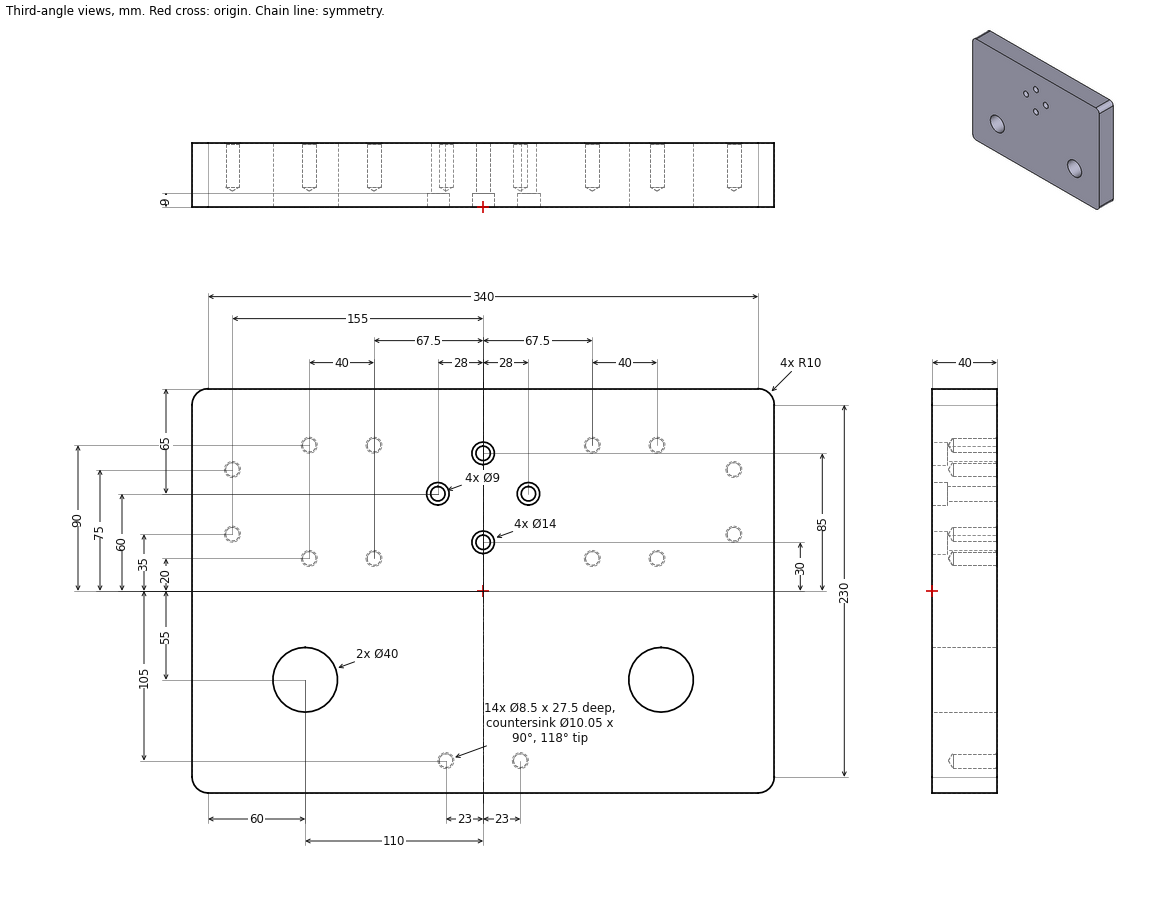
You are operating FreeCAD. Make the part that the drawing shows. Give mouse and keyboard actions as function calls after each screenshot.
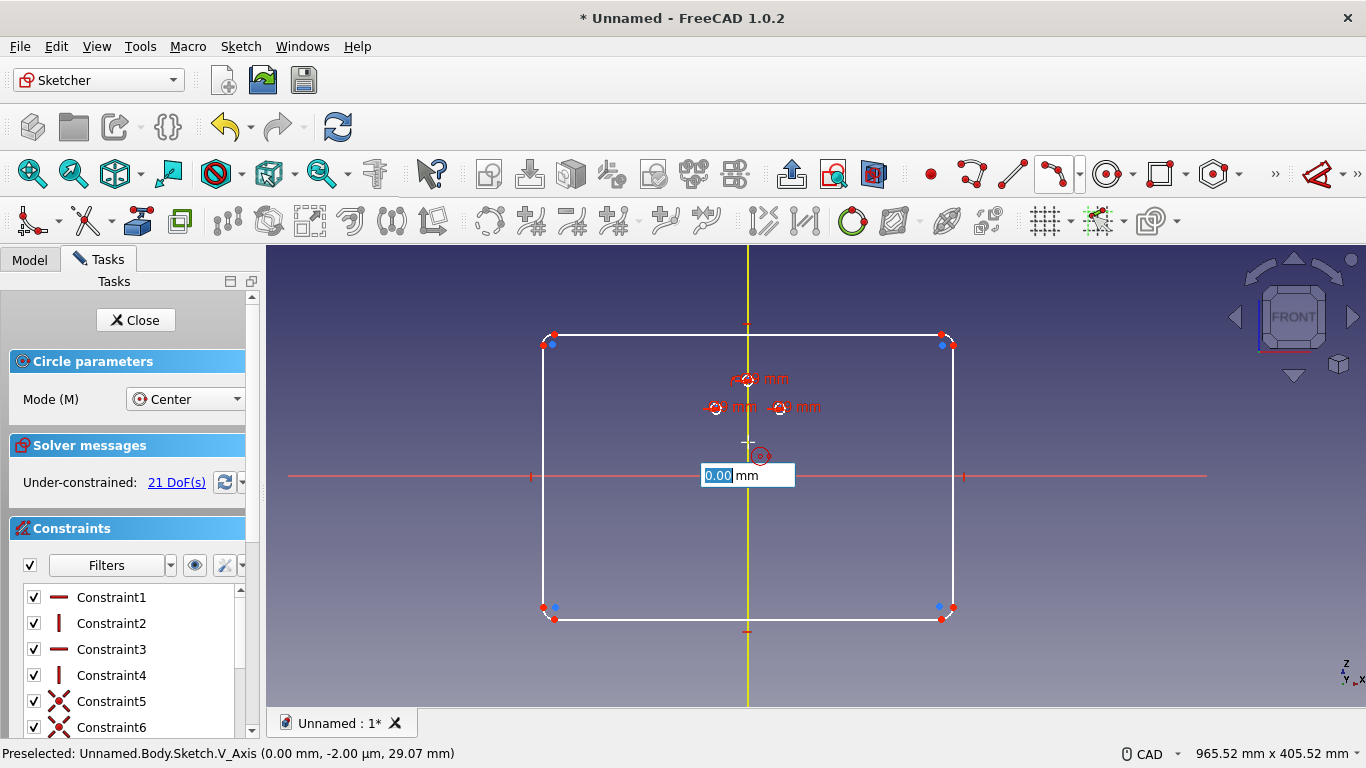
scroll(753, 440, up, 6)
move(751, 440)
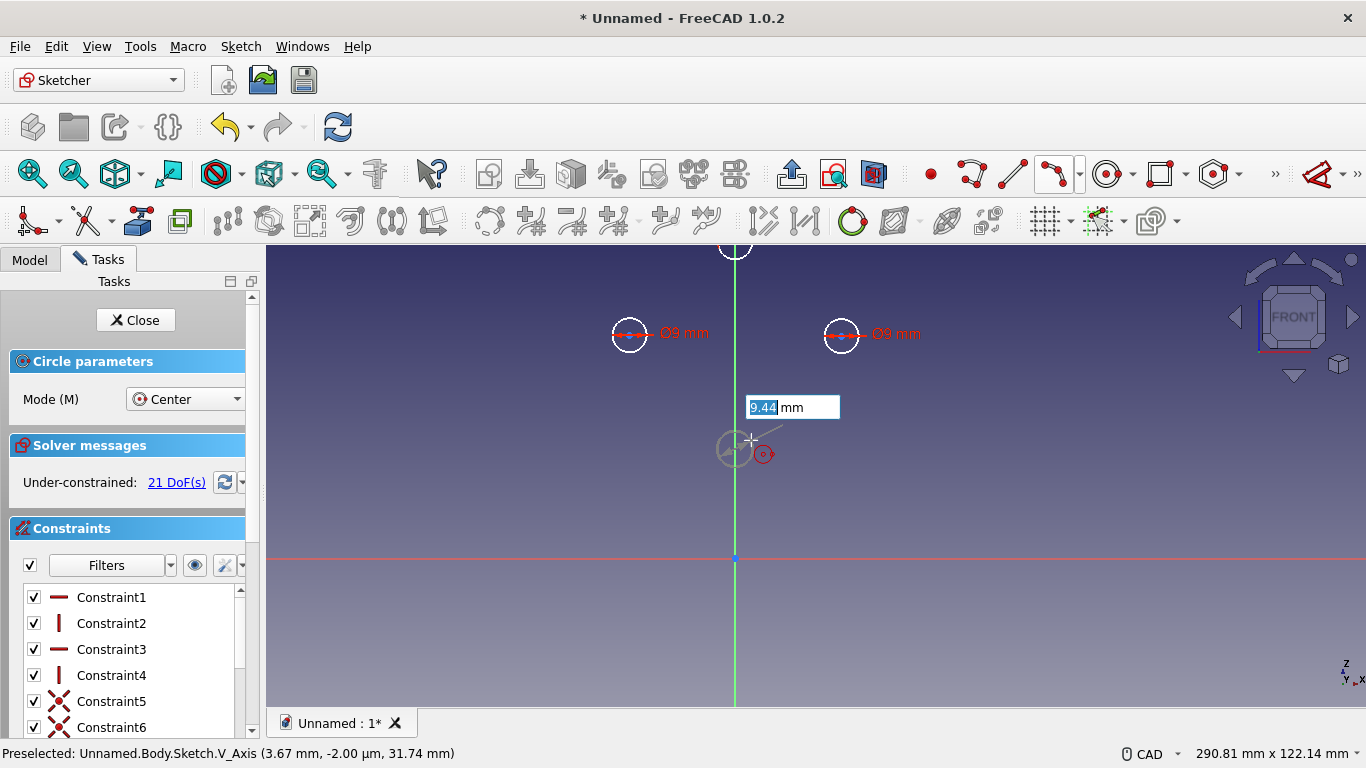
text(9)
key(Return)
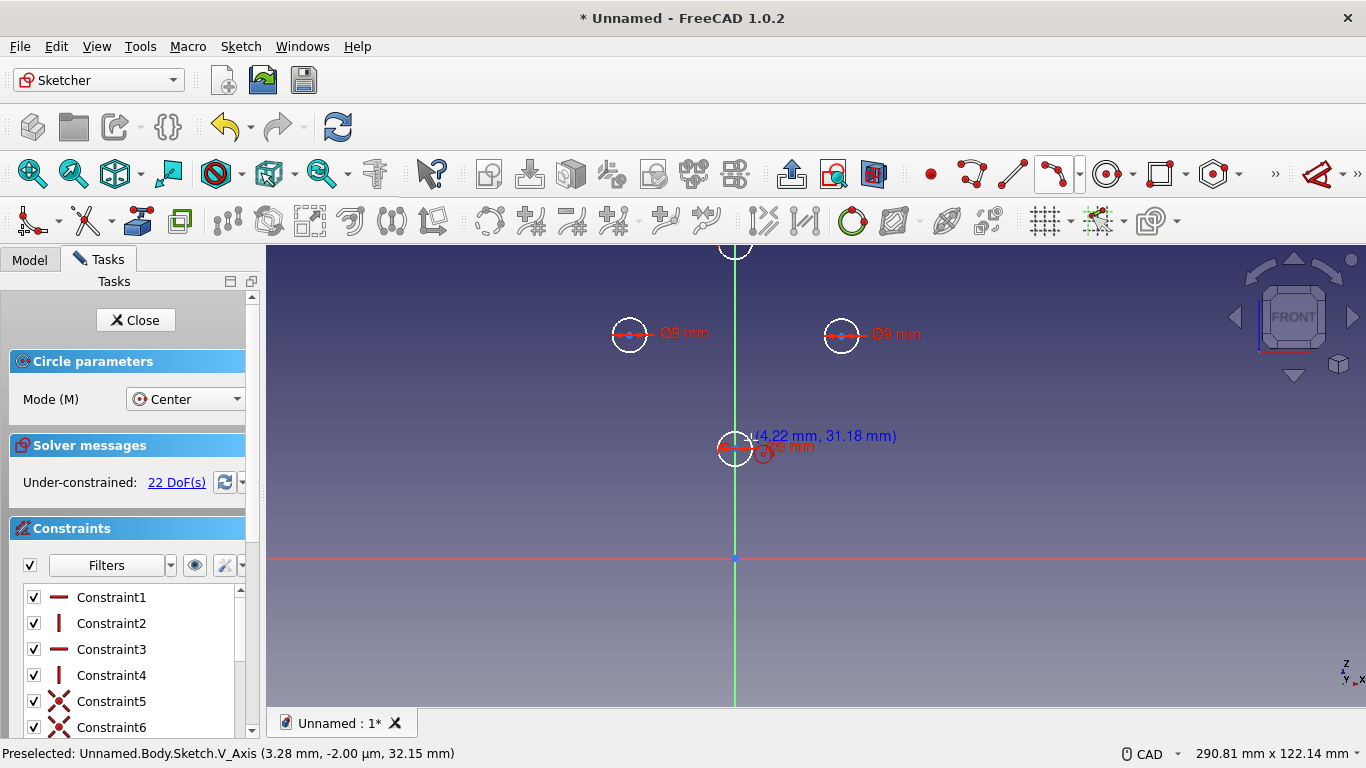
scroll(753, 440, down, 6)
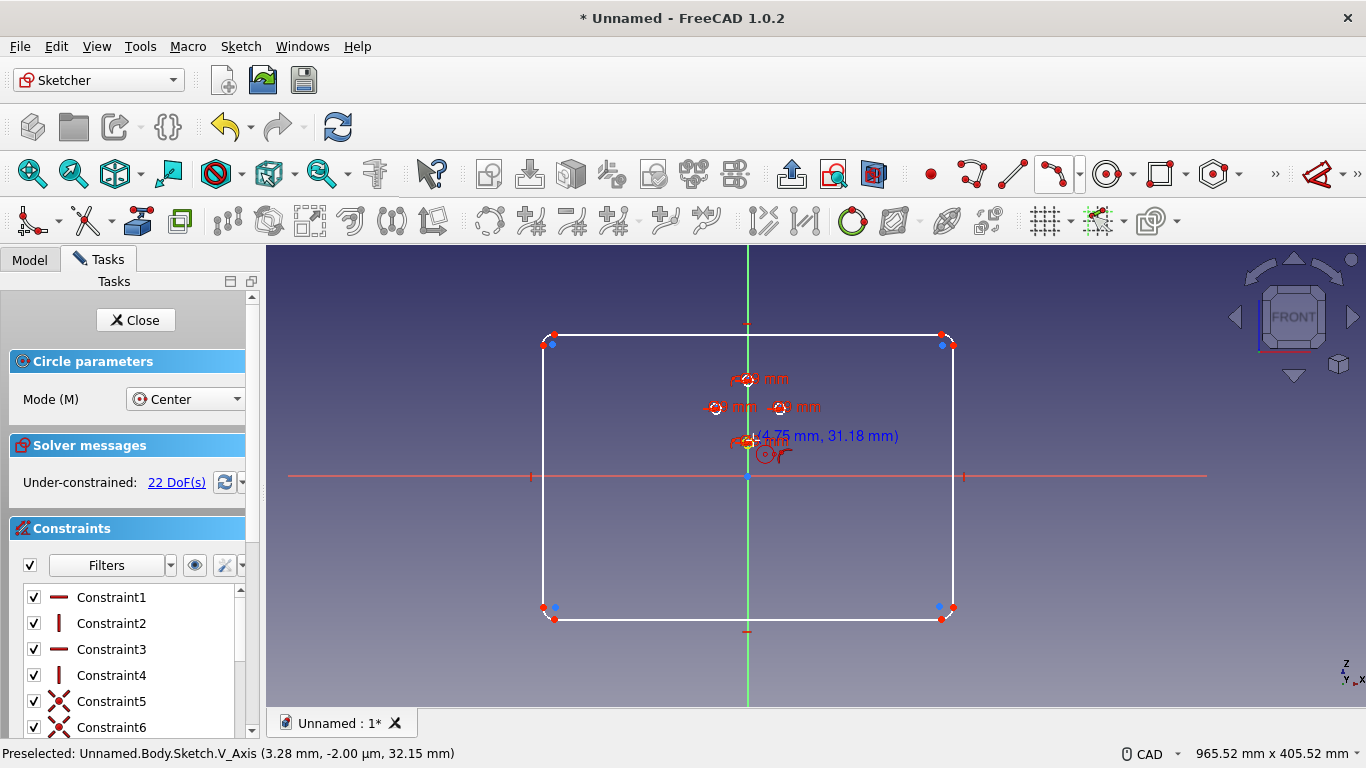
click(623, 539)
move(639, 523)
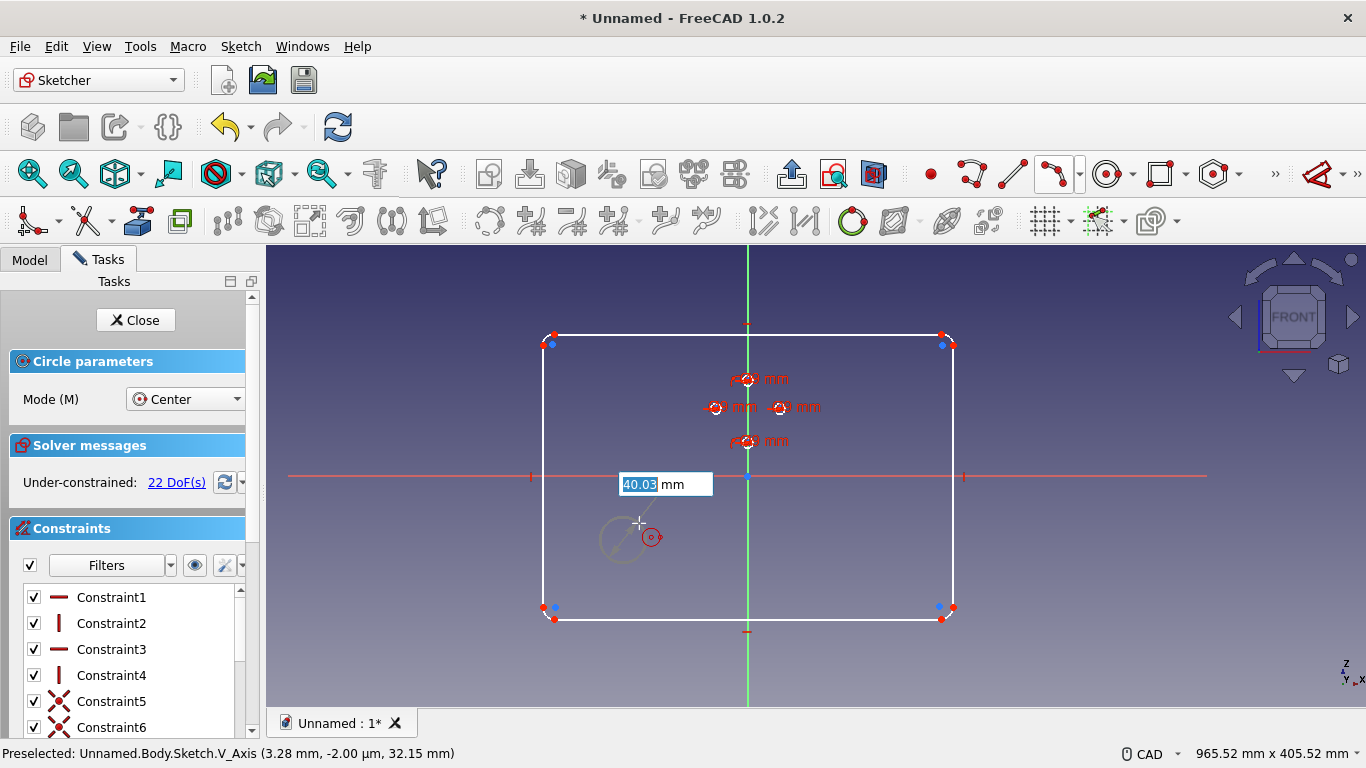
text(40)
key(Return)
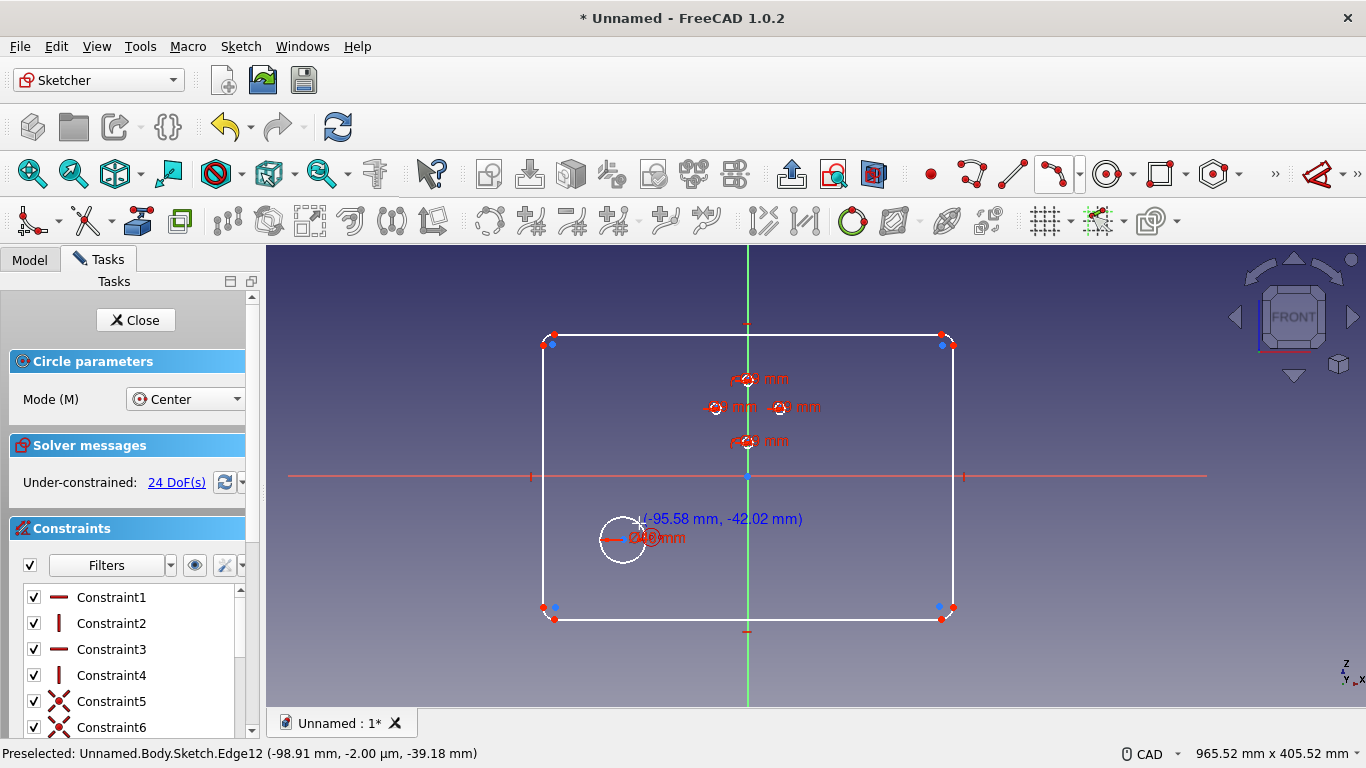
click(873, 539)
move(889, 523)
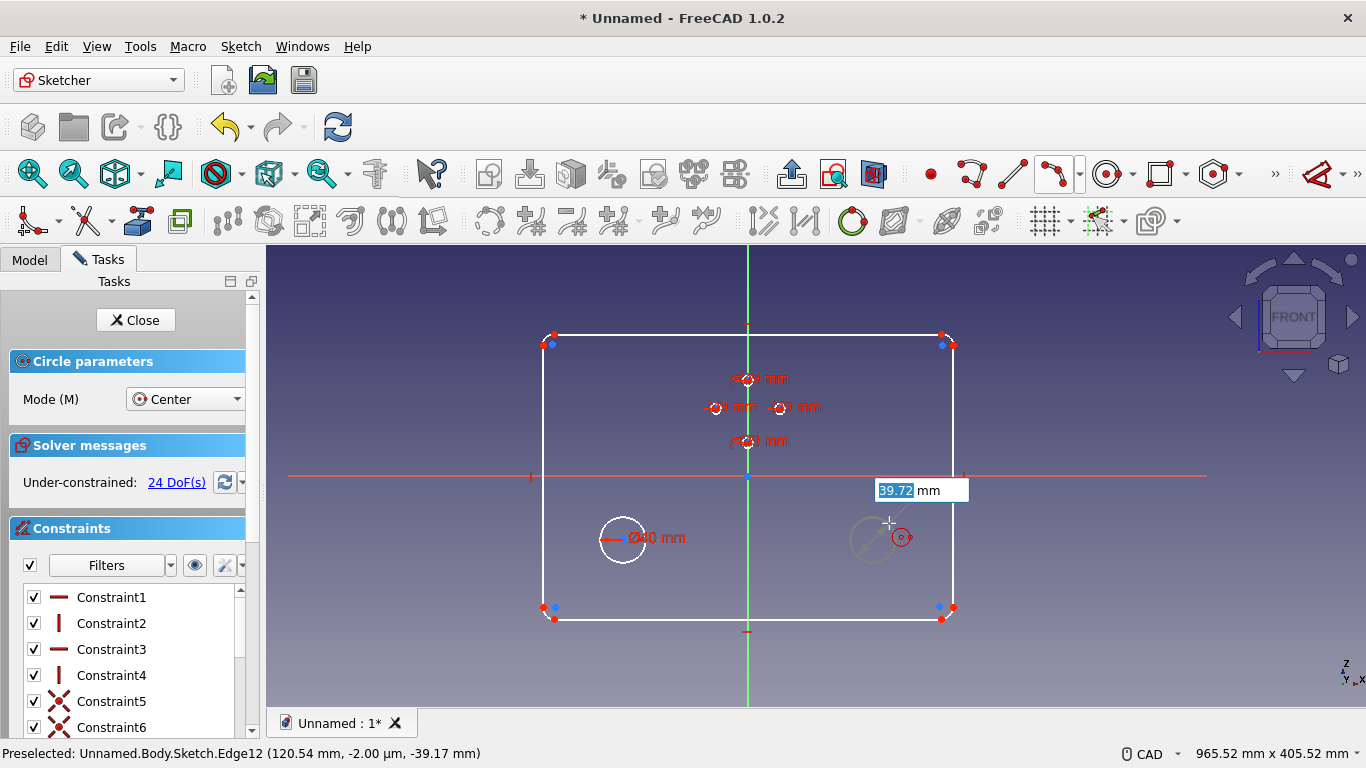
text(40)
key(Return)
key(Escape)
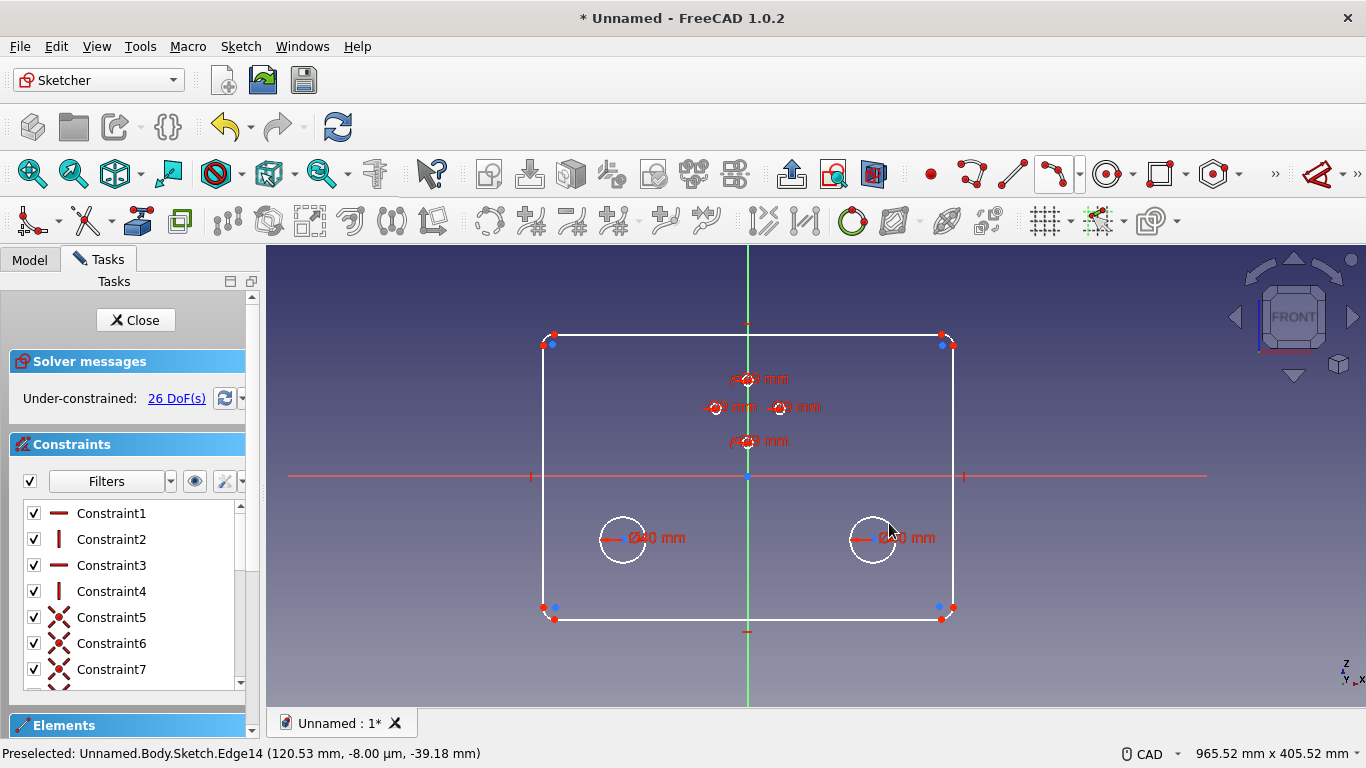
click(670, 335)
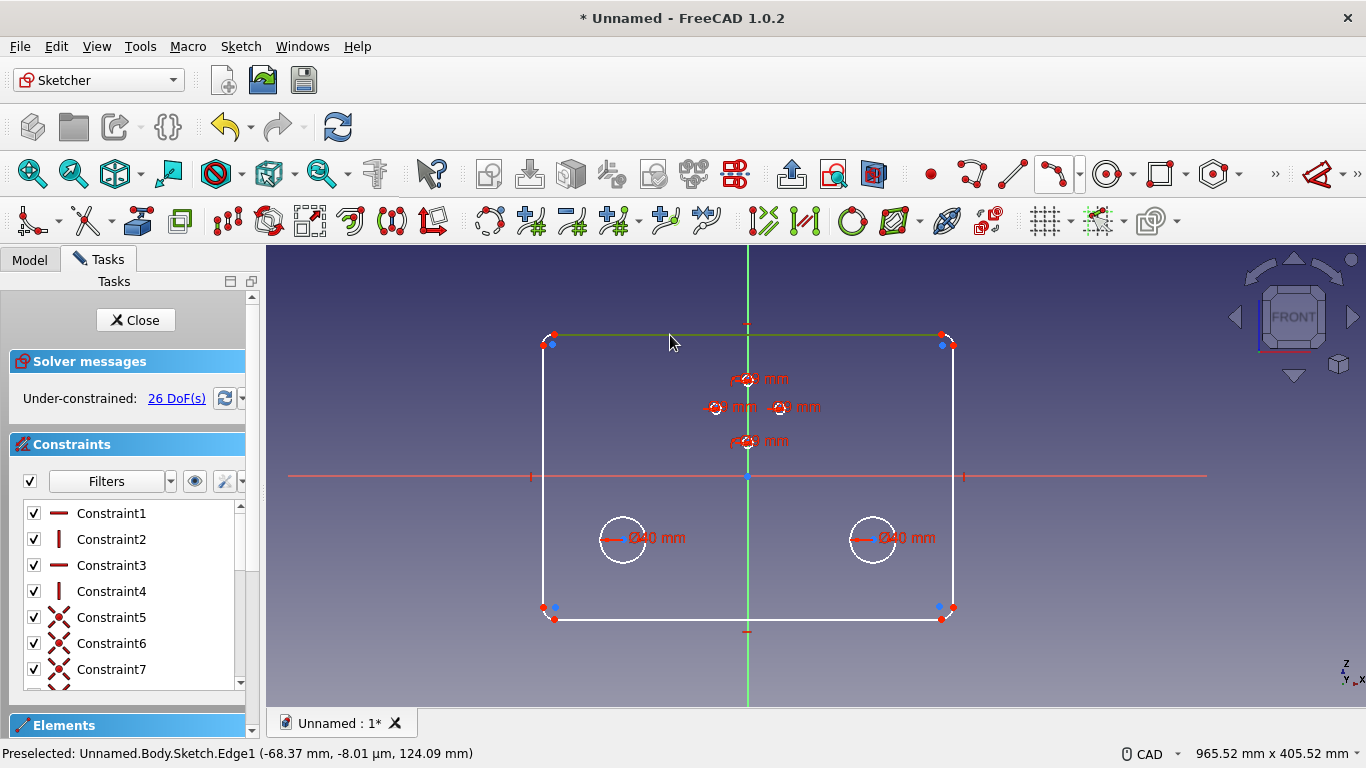
scroll(950, 337, up, 3)